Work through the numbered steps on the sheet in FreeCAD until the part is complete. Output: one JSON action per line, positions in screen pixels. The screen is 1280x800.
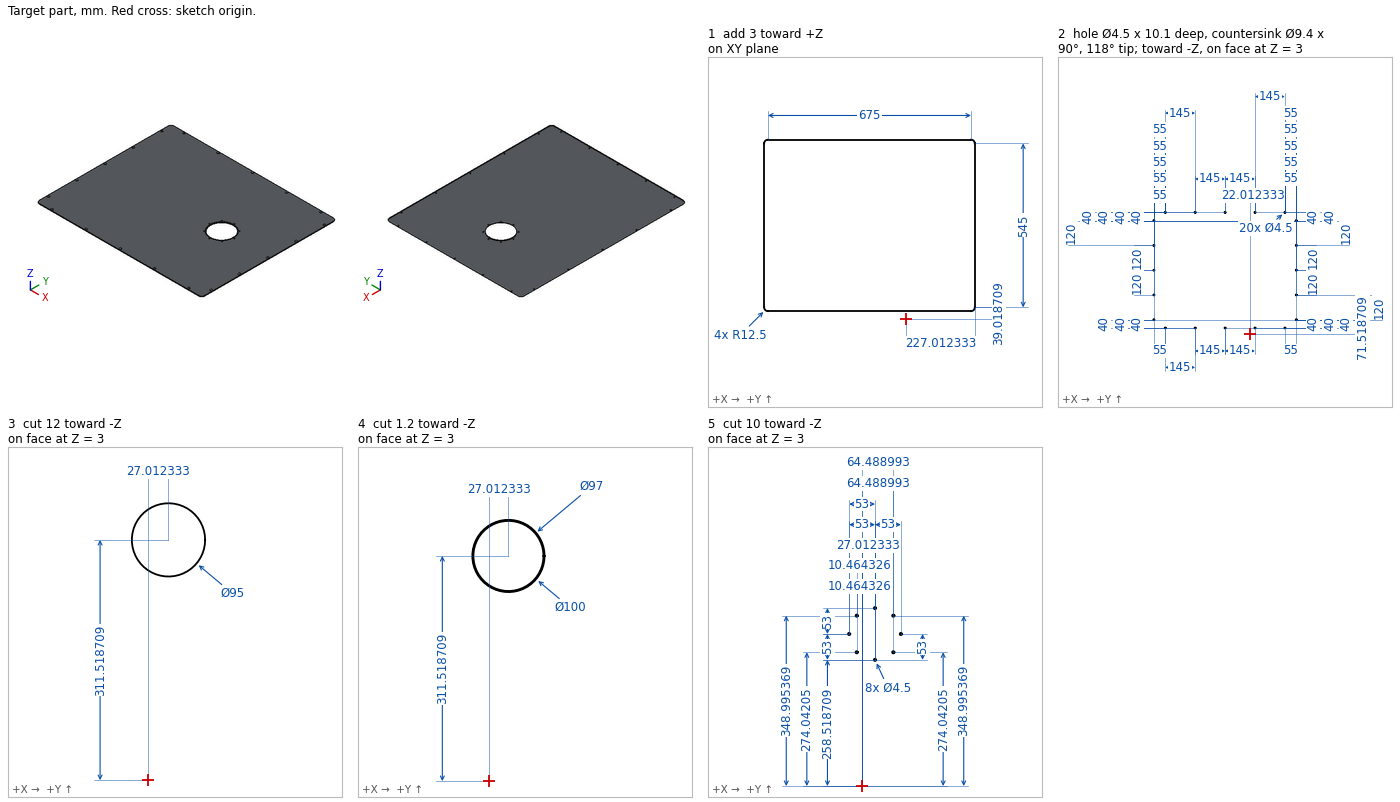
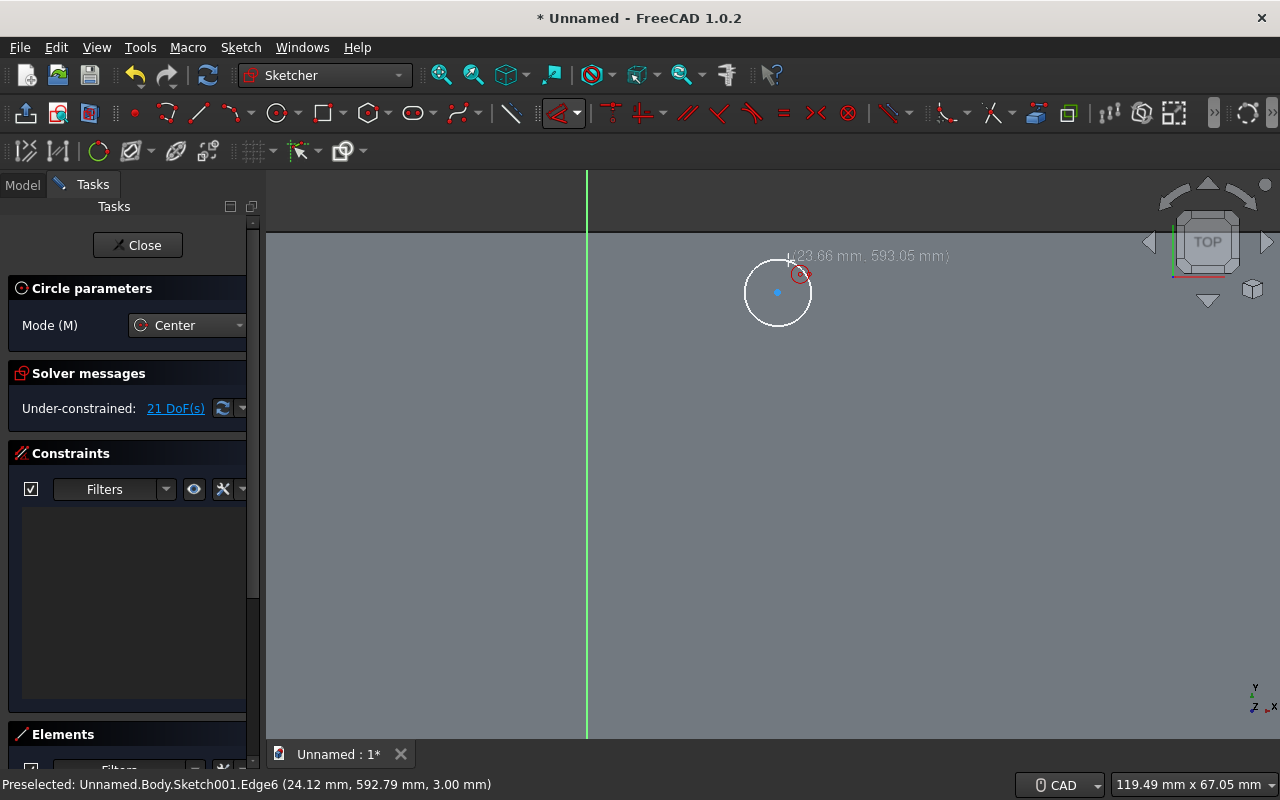
{"action": "scroll", "coordinate": [798, 268], "scroll_direction": "down", "scroll_amount": 13}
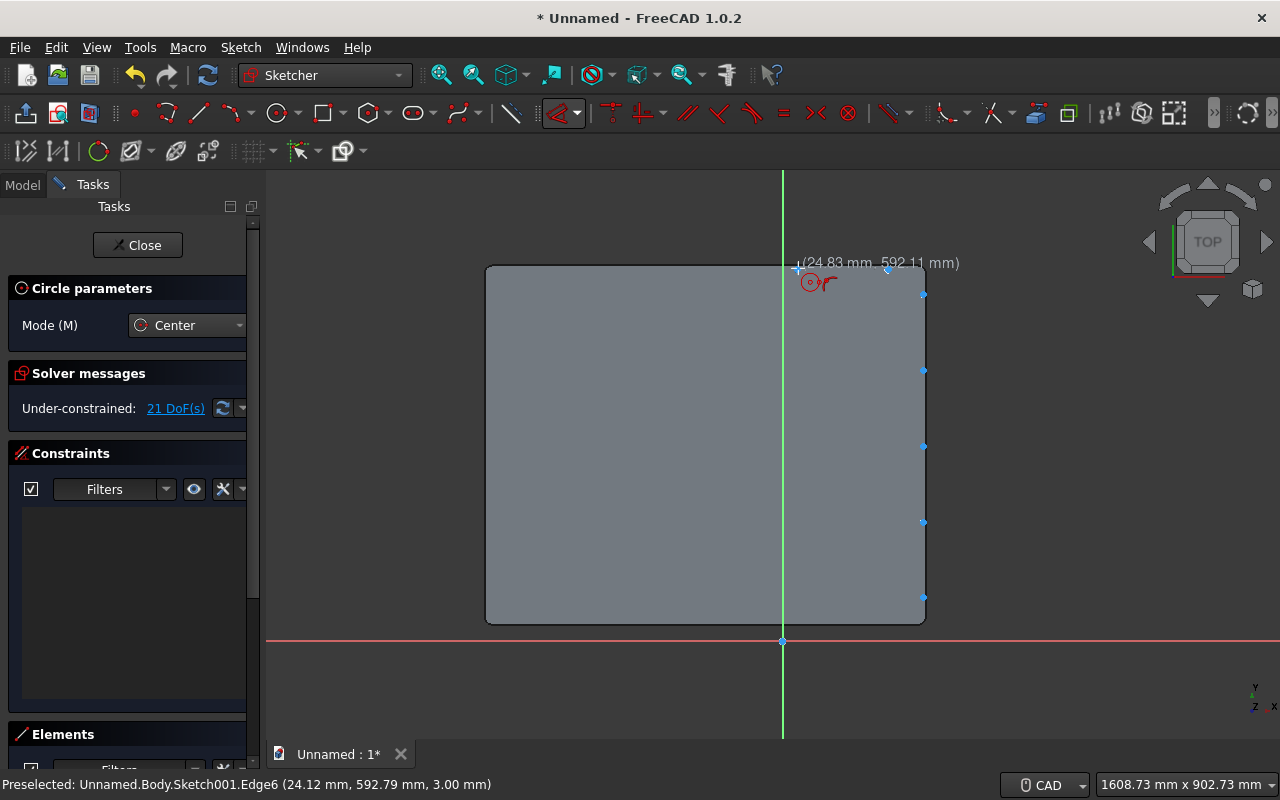
{"action": "scroll", "coordinate": [705, 269], "scroll_direction": "up", "scroll_amount": 14}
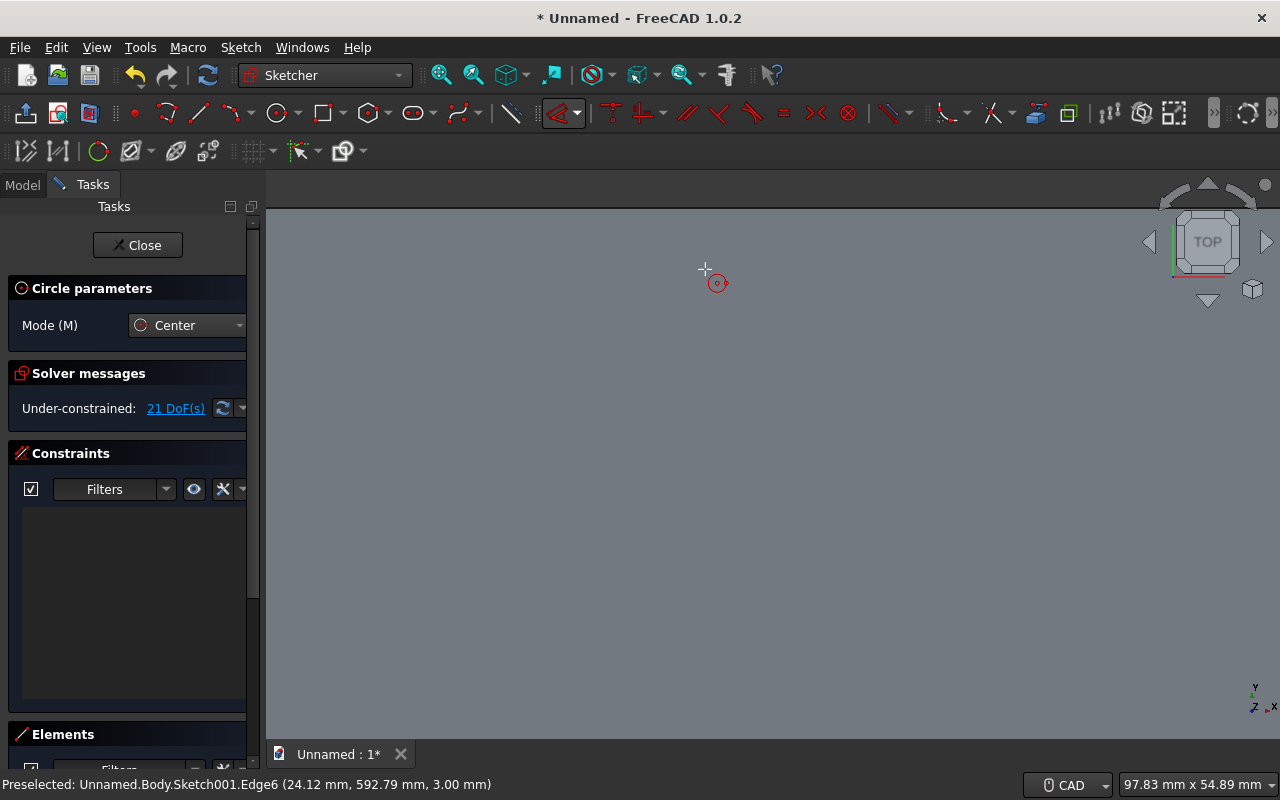
{"action": "scroll", "coordinate": [705, 269], "scroll_direction": "down", "scroll_amount": 14}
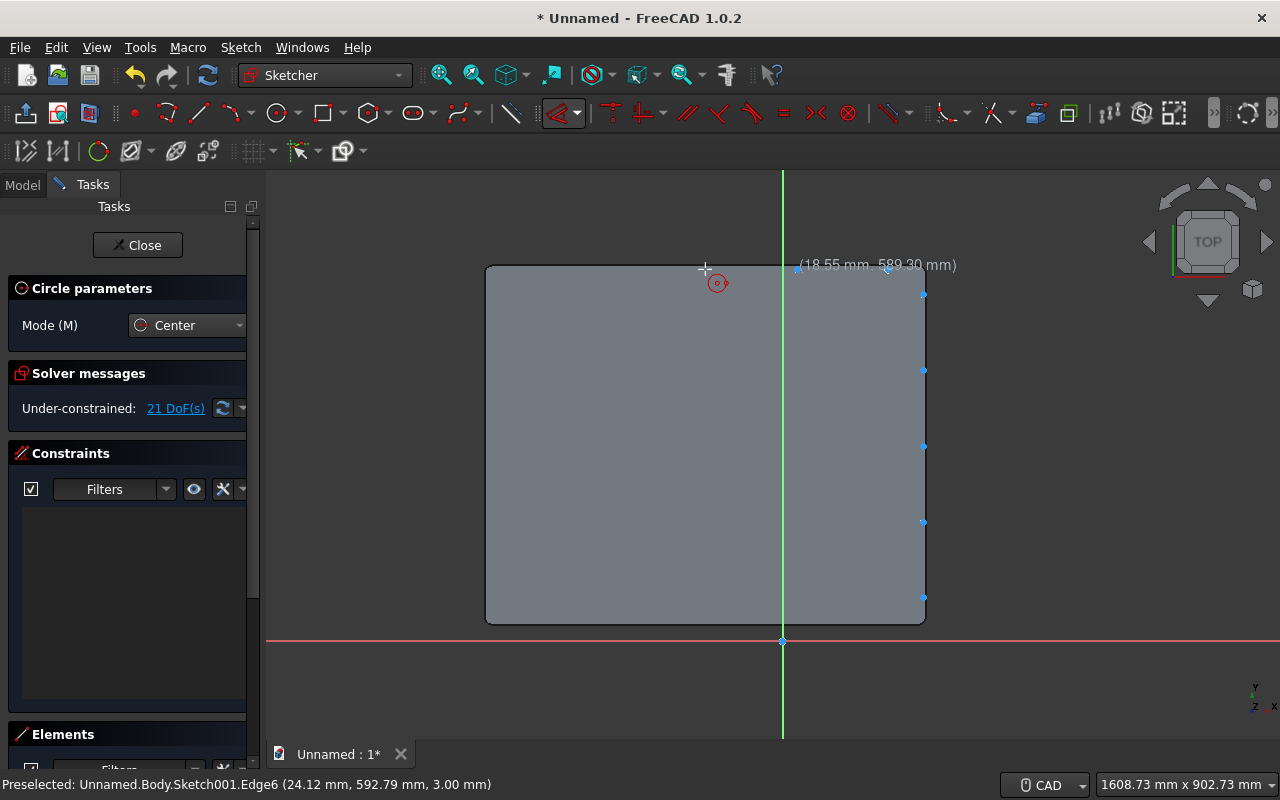
{"action": "left_click", "coordinate": [705, 269]}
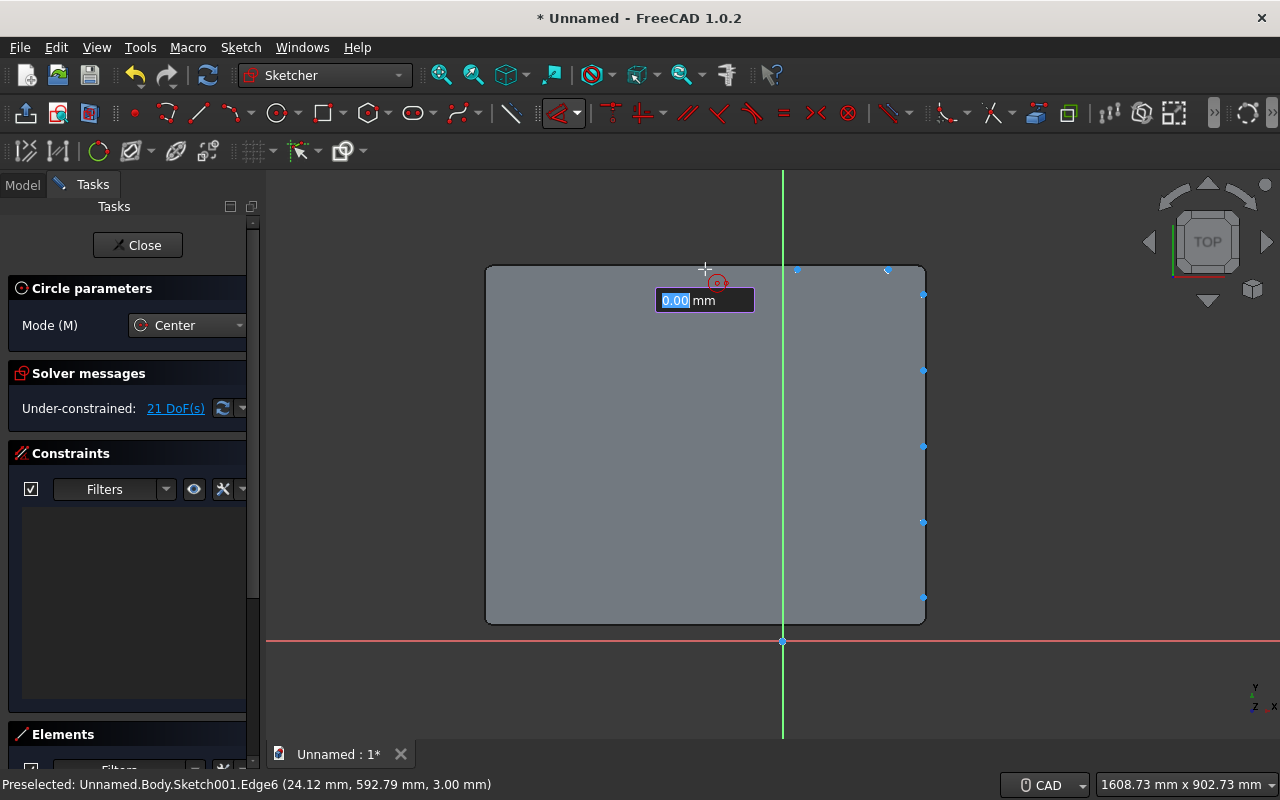
{"action": "scroll", "coordinate": [706, 268], "scroll_direction": "up", "scroll_amount": 13}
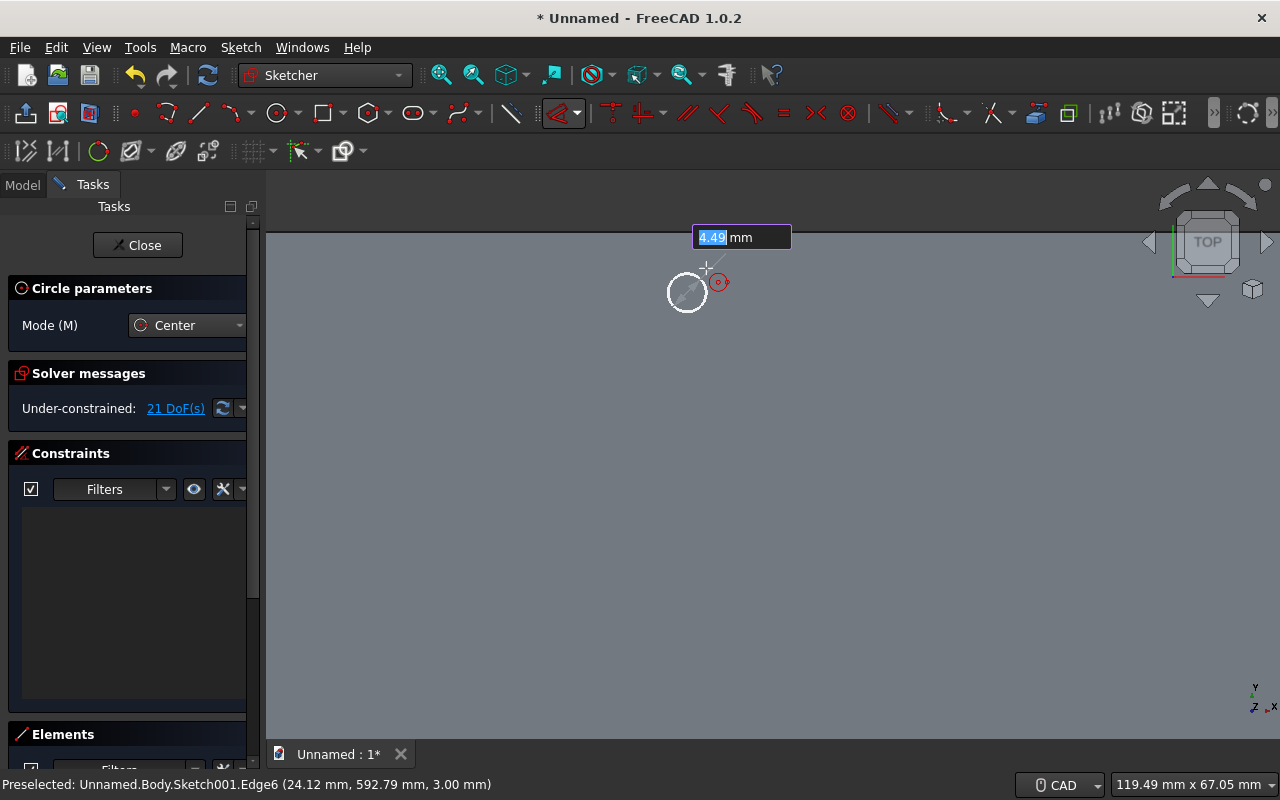
{"action": "left_click", "coordinate": [705, 260]}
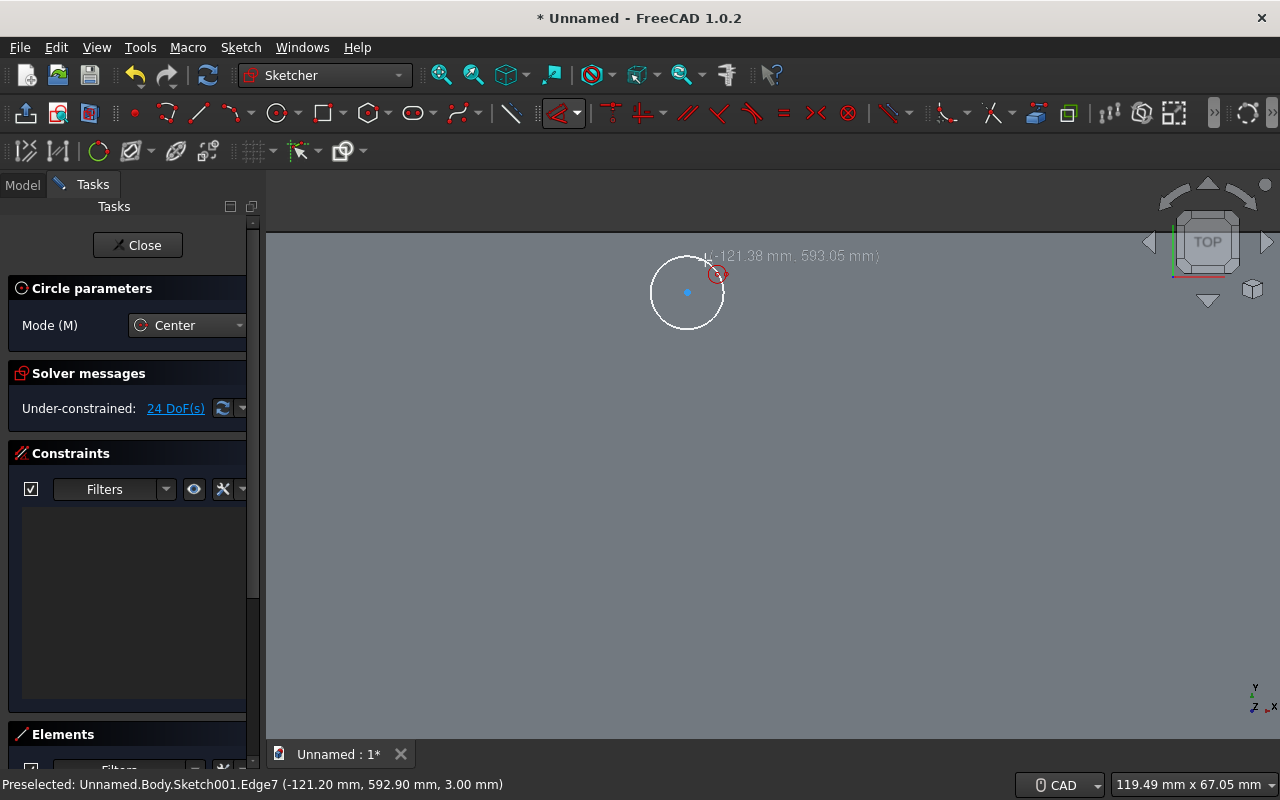
{"action": "scroll", "coordinate": [706, 268], "scroll_direction": "down", "scroll_amount": 13}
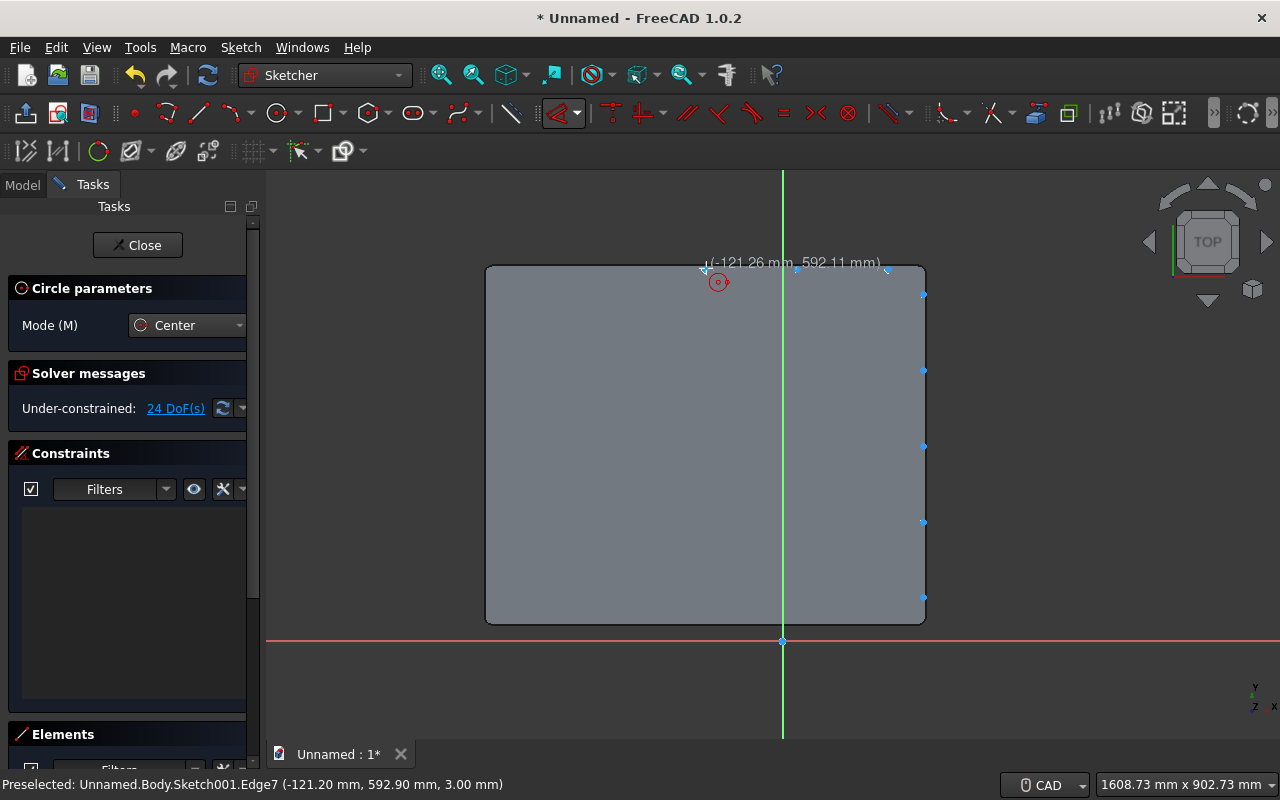
{"action": "scroll", "coordinate": [614, 269], "scroll_direction": "up", "scroll_amount": 14}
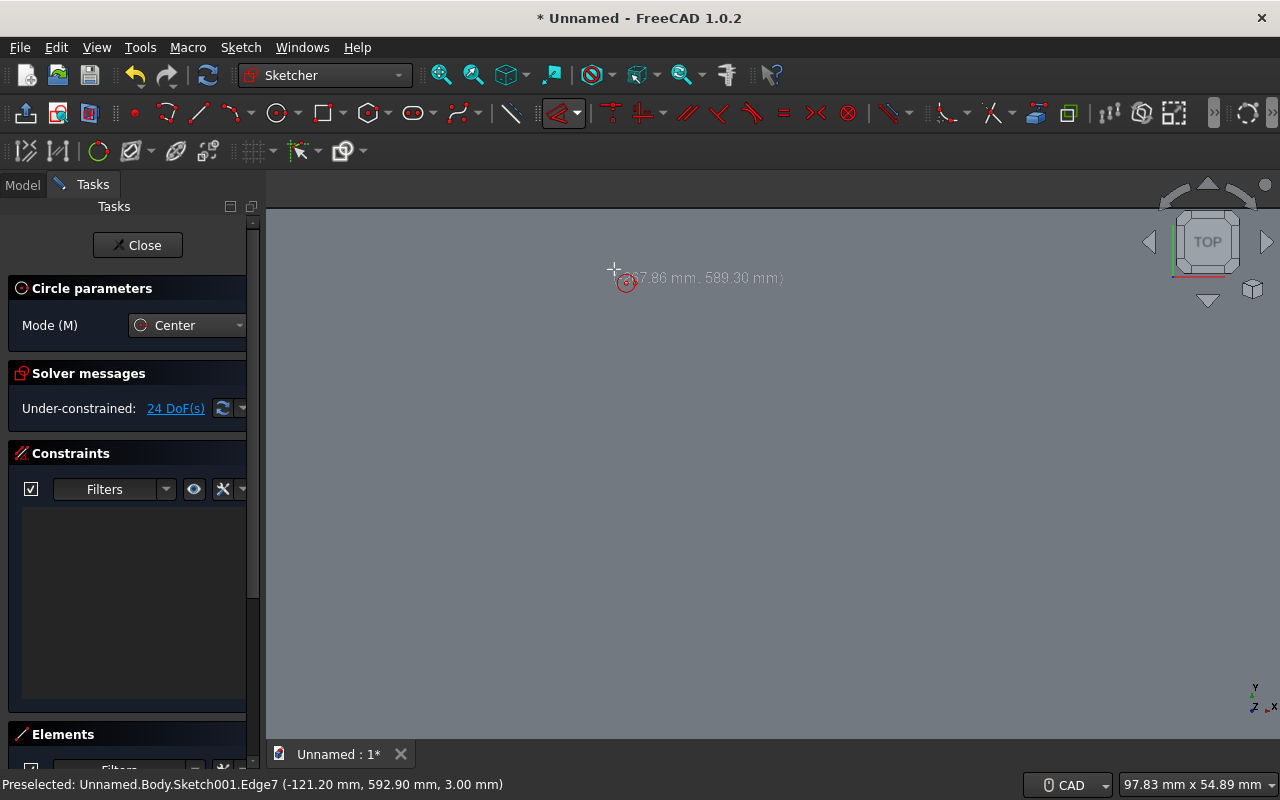
{"action": "scroll", "coordinate": [613, 269], "scroll_direction": "down", "scroll_amount": 14}